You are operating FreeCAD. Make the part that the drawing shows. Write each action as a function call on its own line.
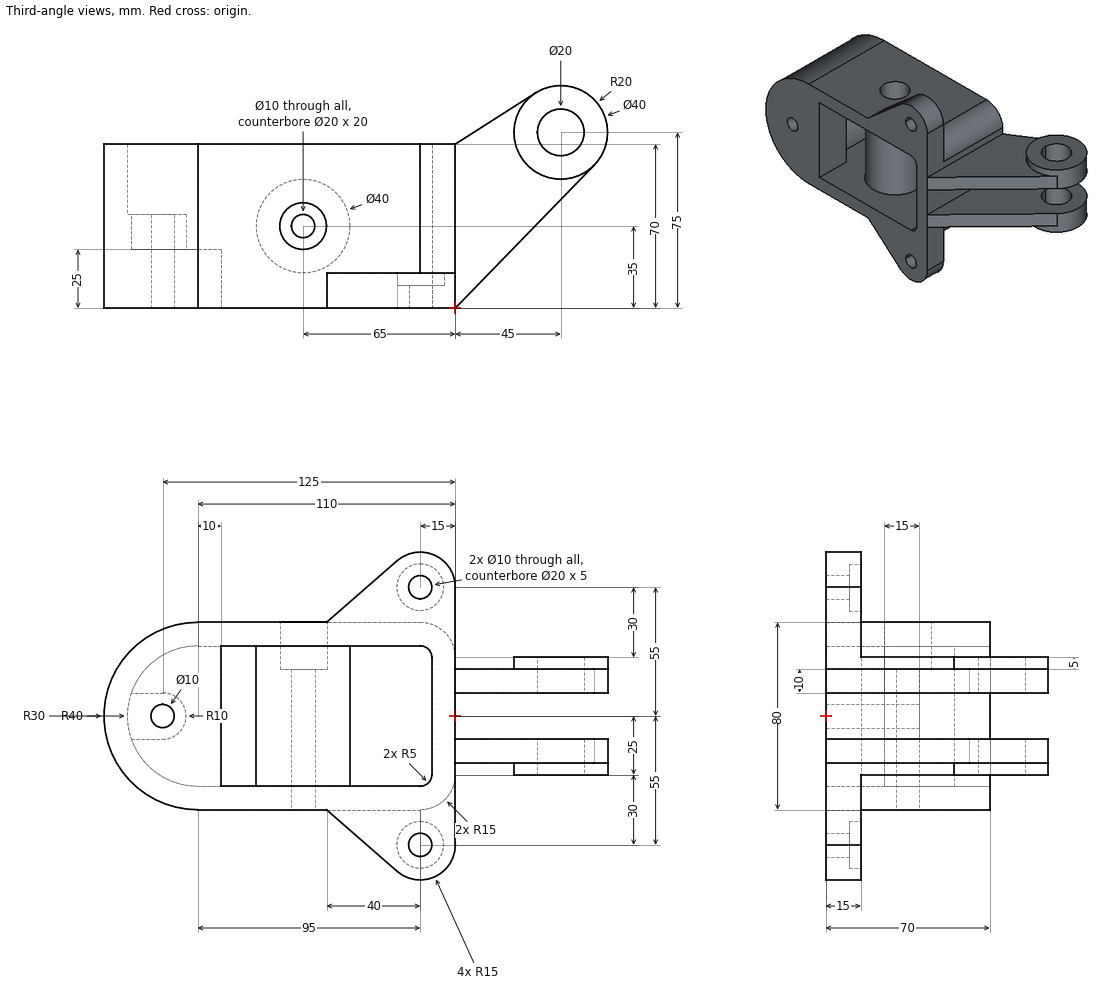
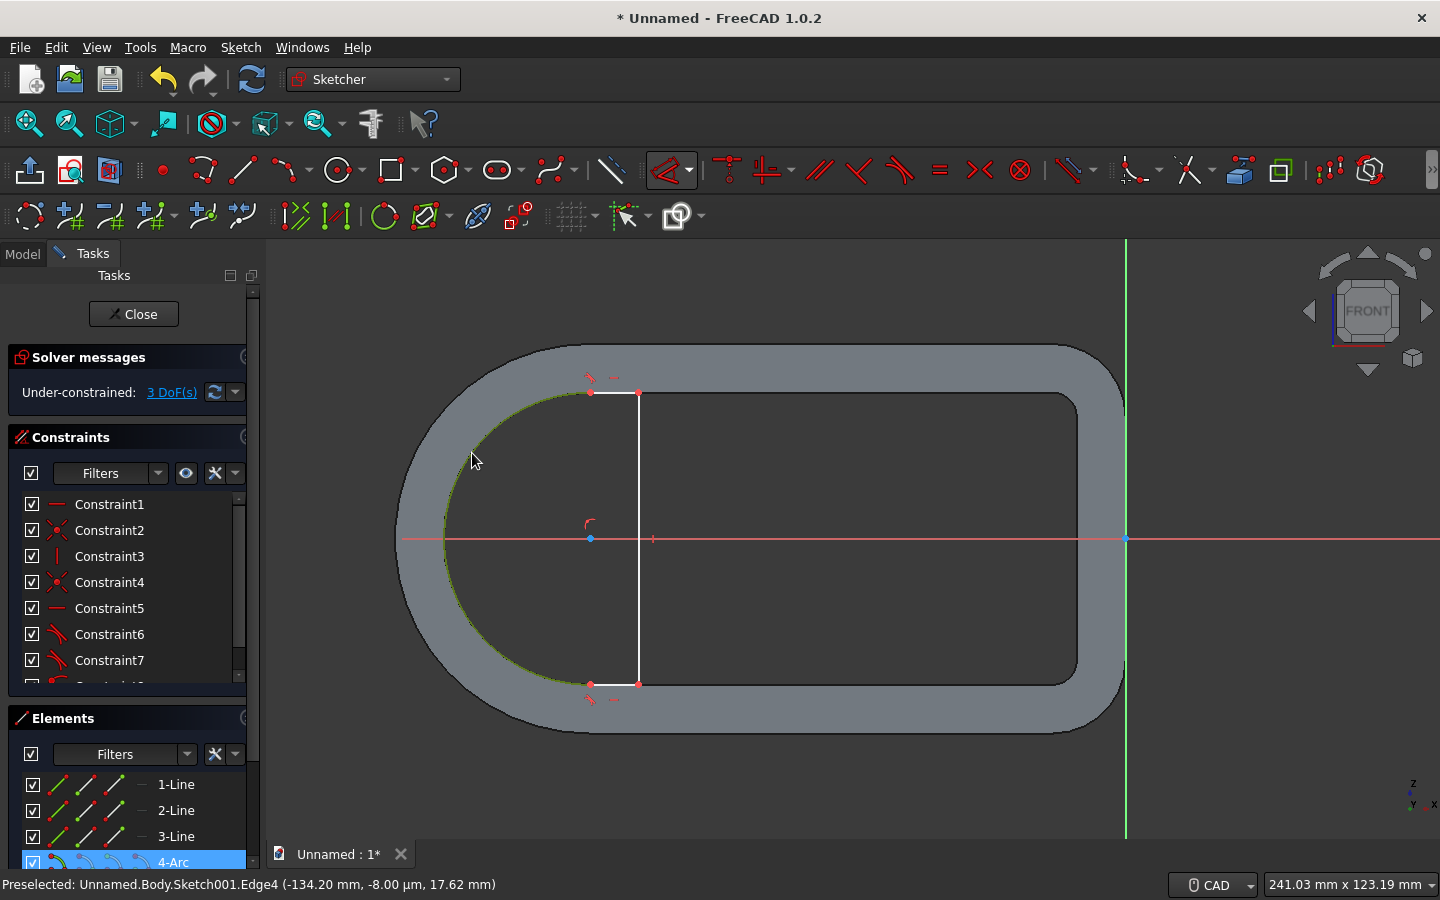
key(k)
key(r)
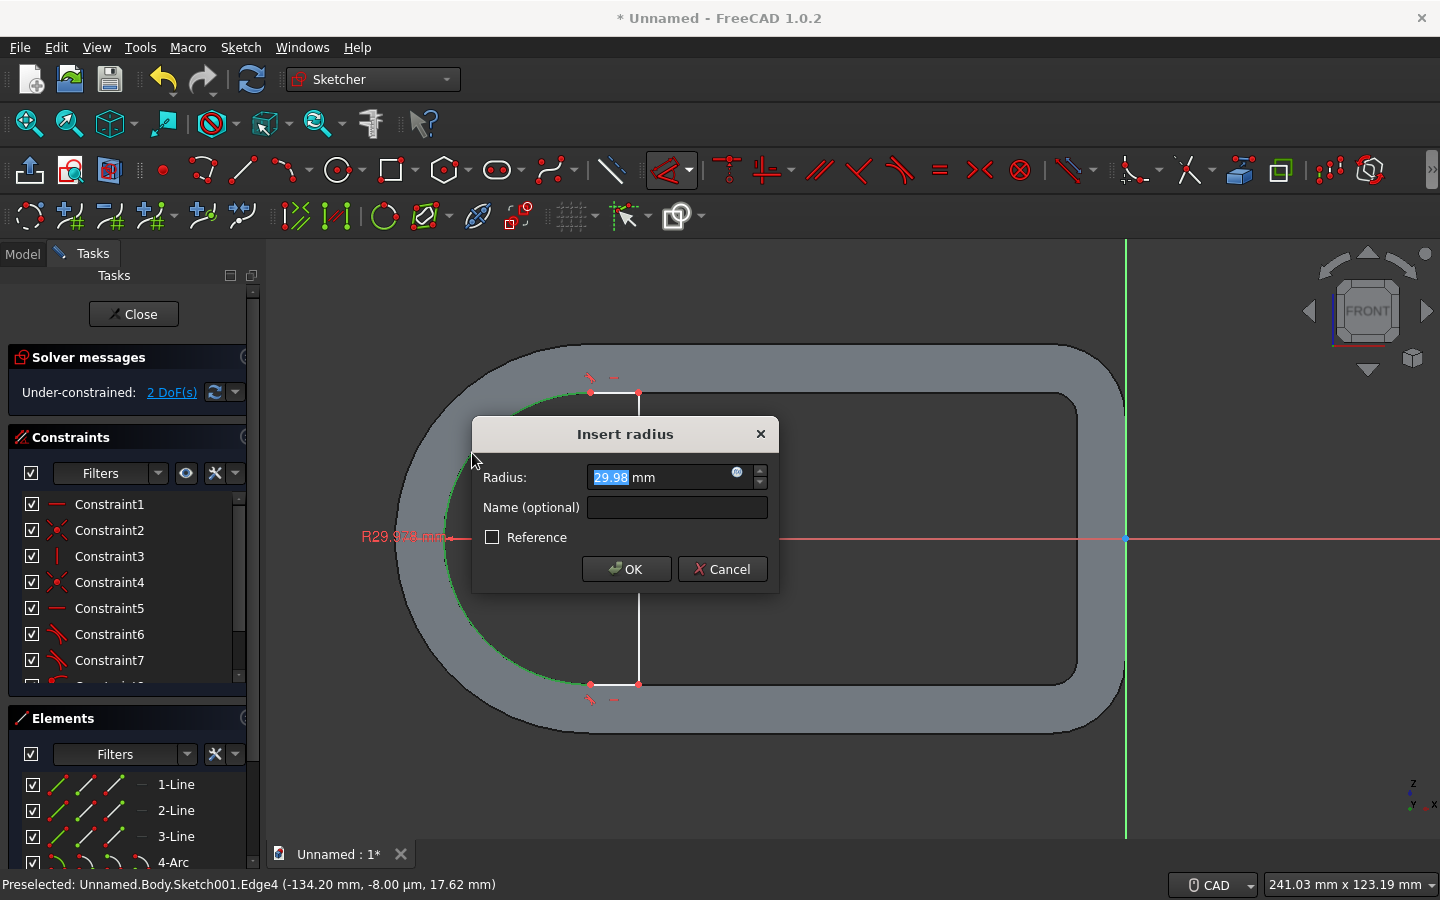
text(30)
key(Return)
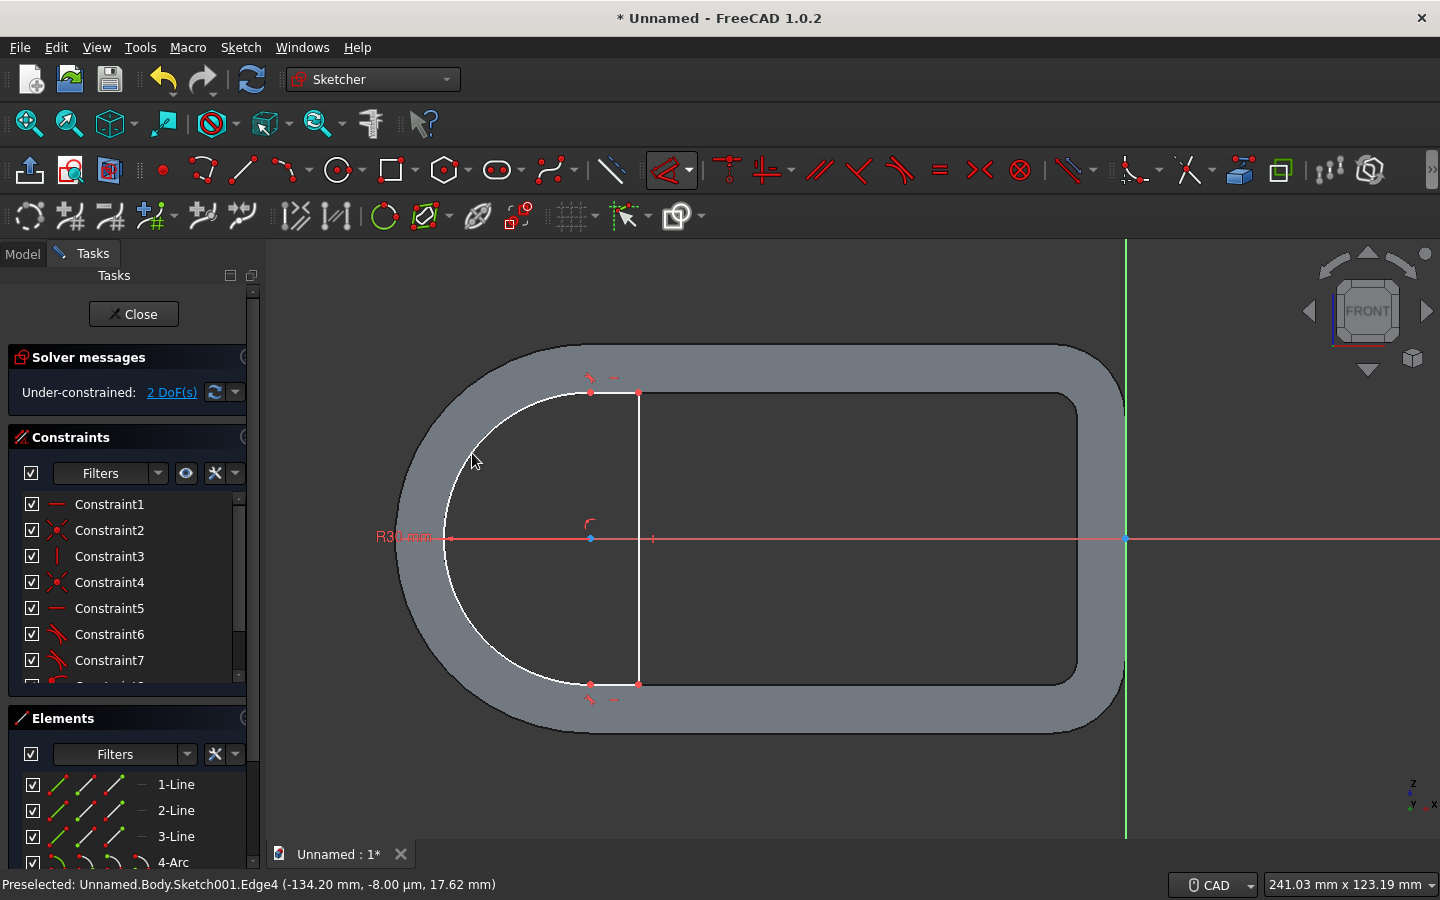
click(605, 393)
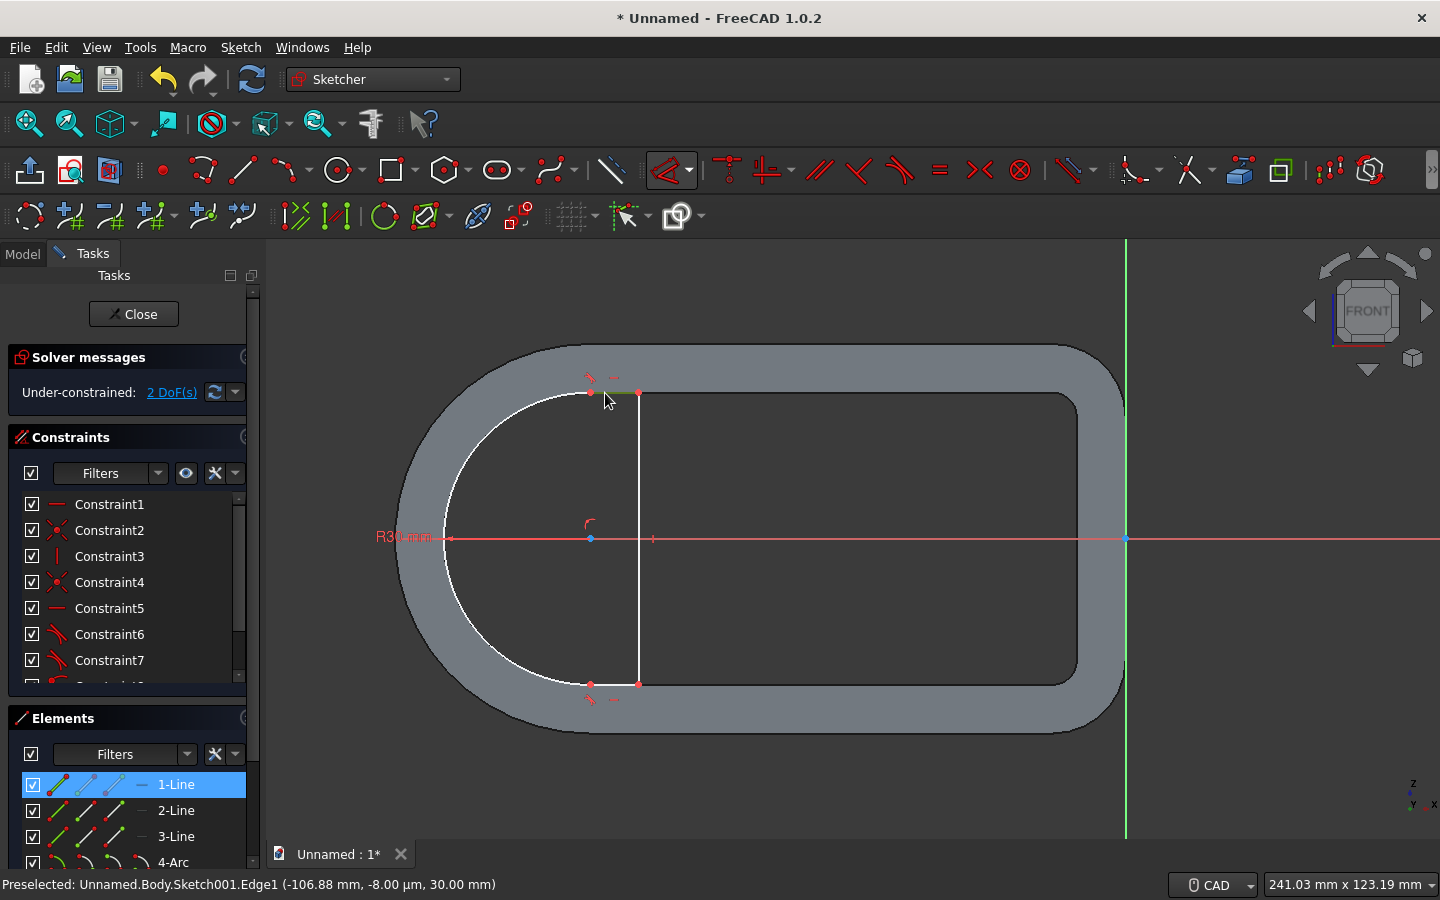
key(l)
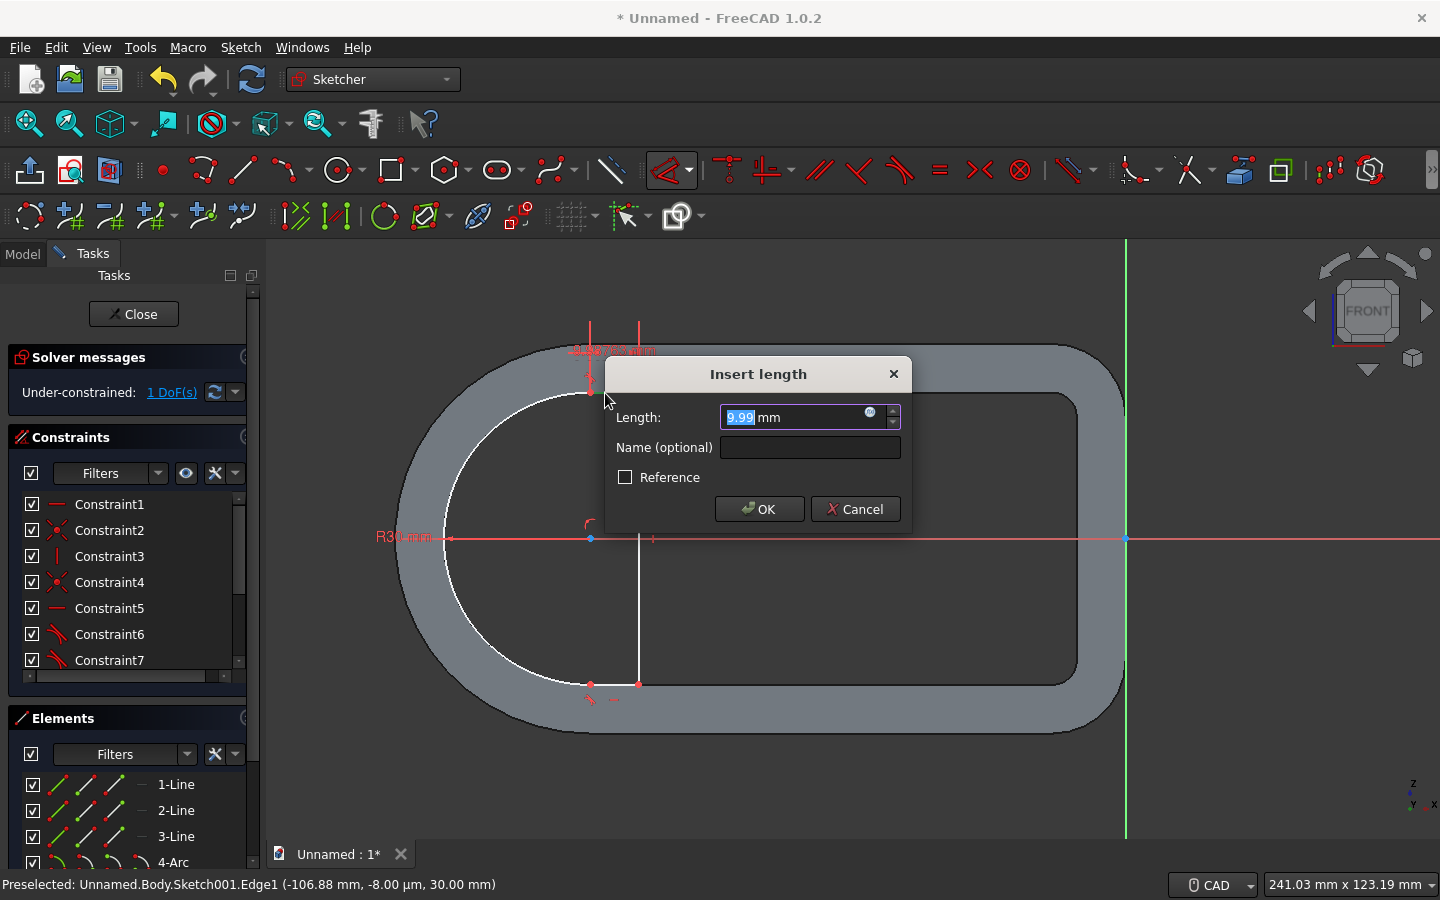
text(10)
key(Return)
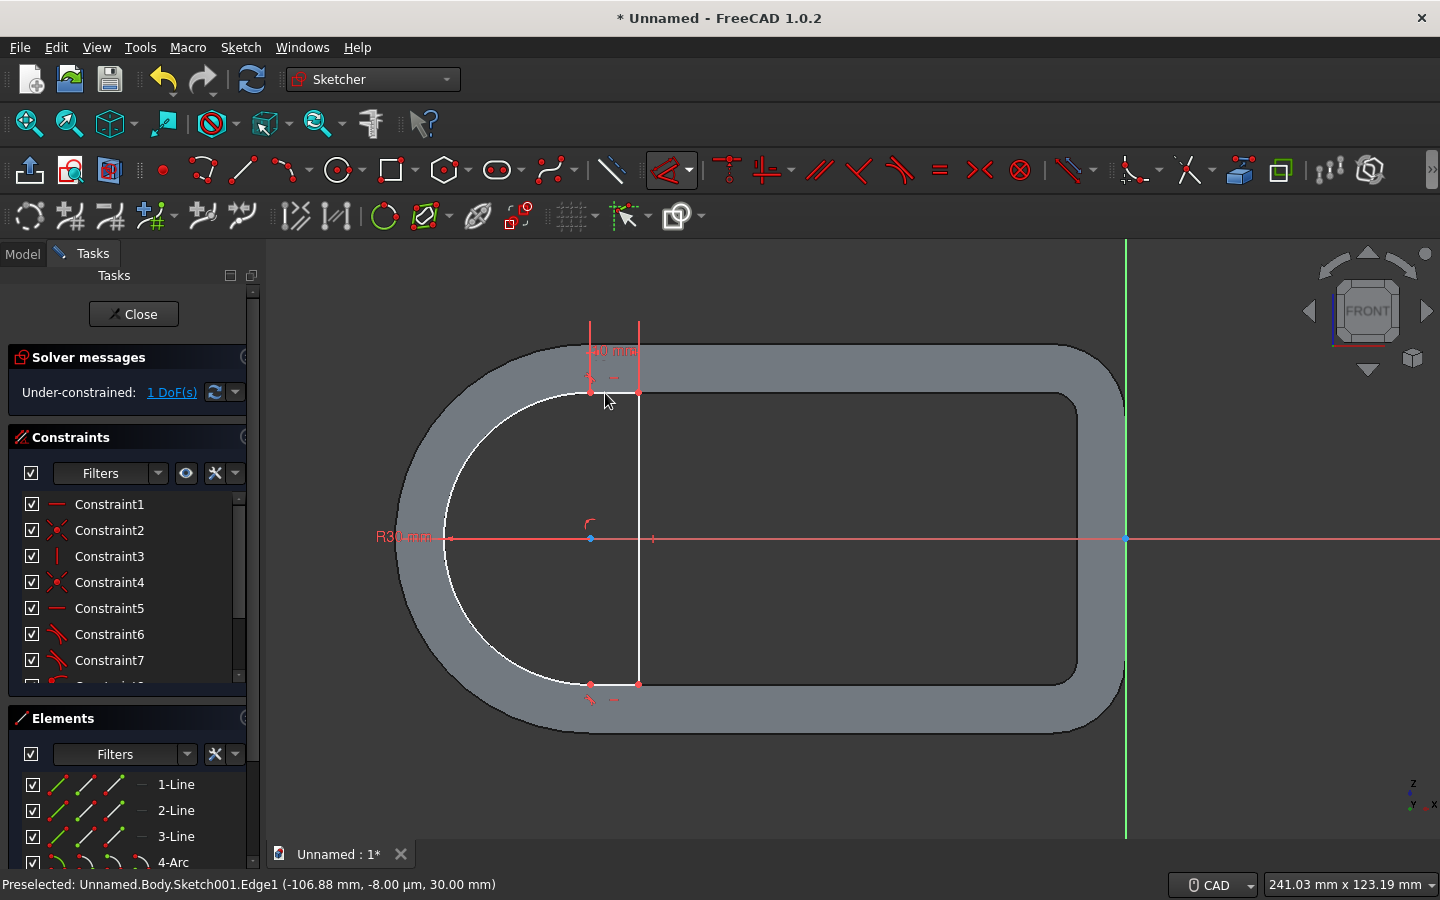
click(590, 393)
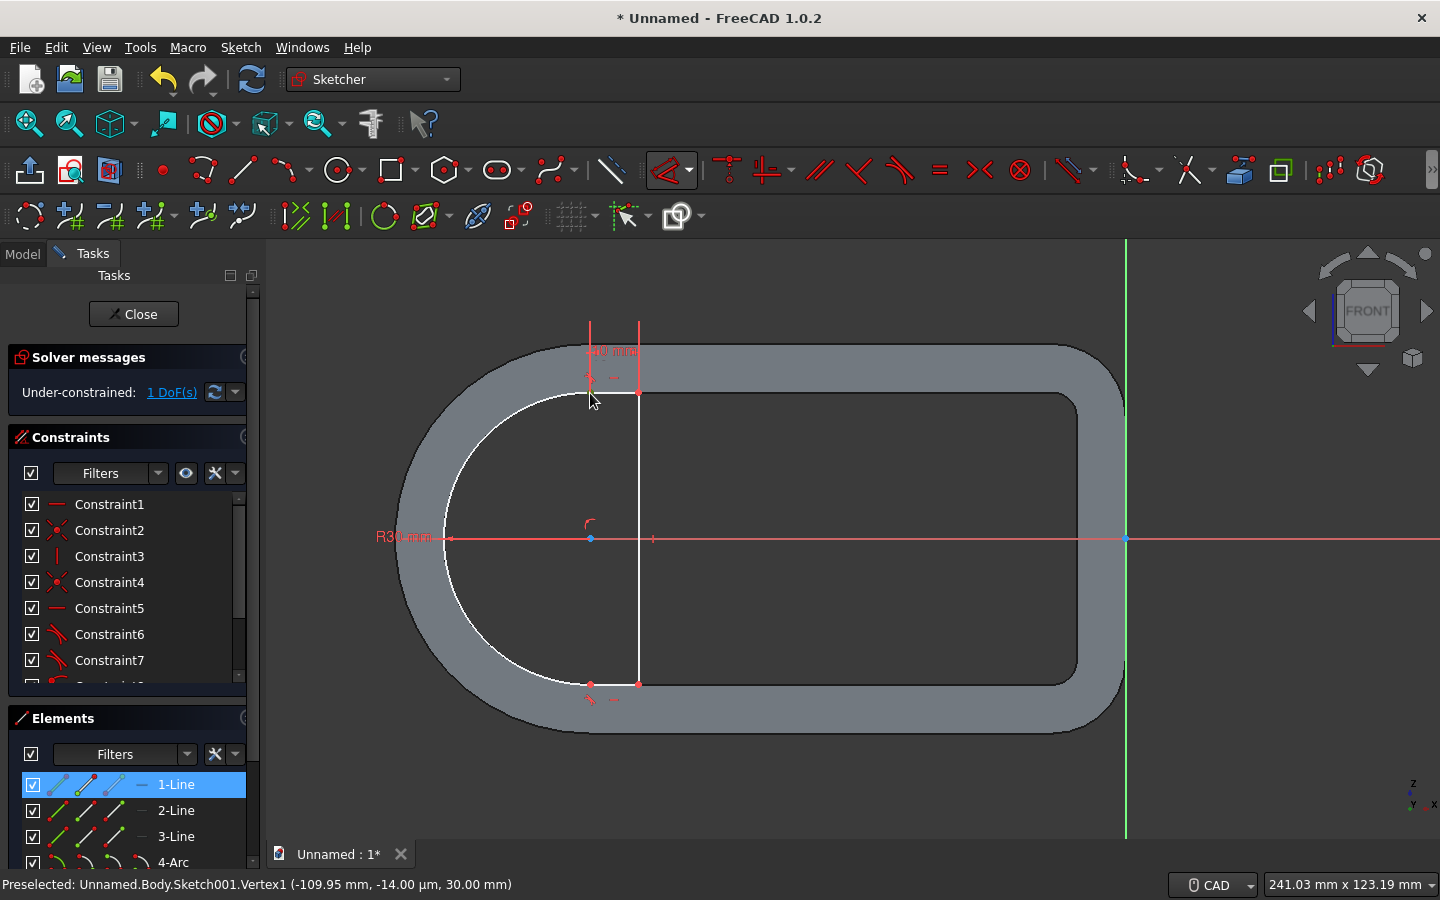
key(l)